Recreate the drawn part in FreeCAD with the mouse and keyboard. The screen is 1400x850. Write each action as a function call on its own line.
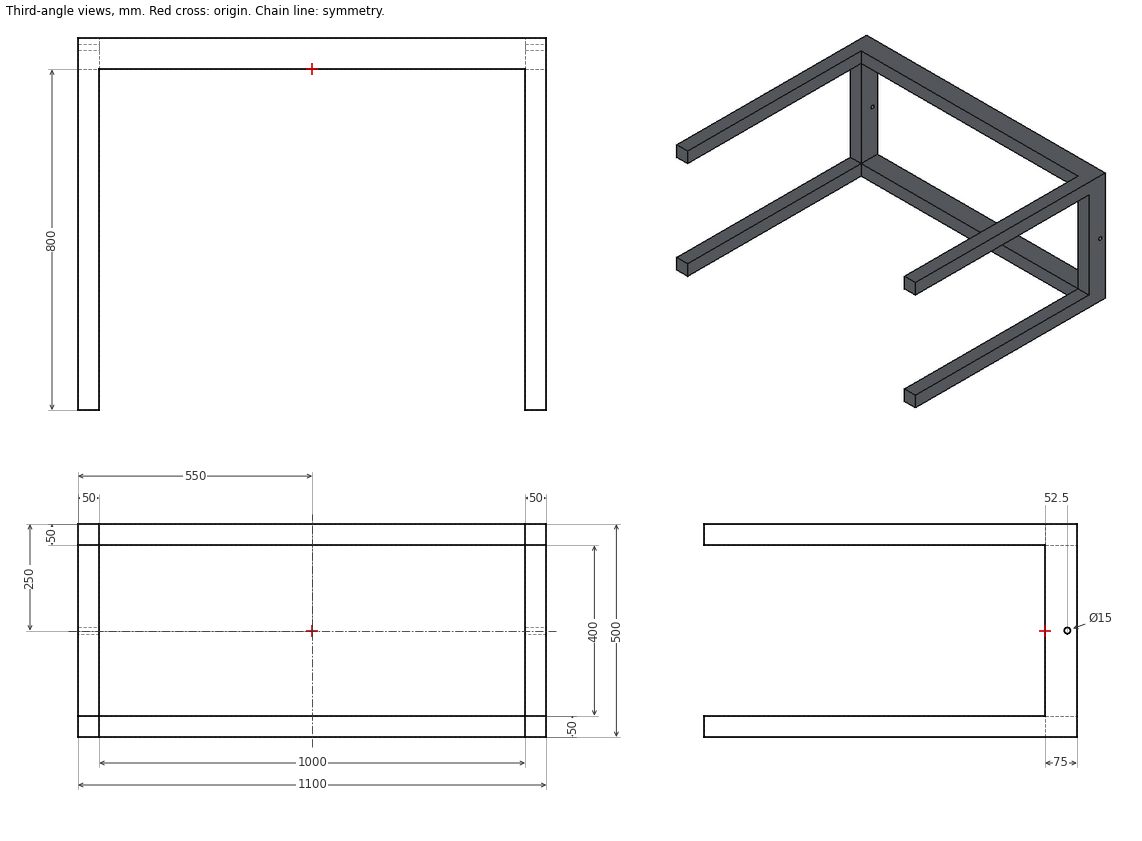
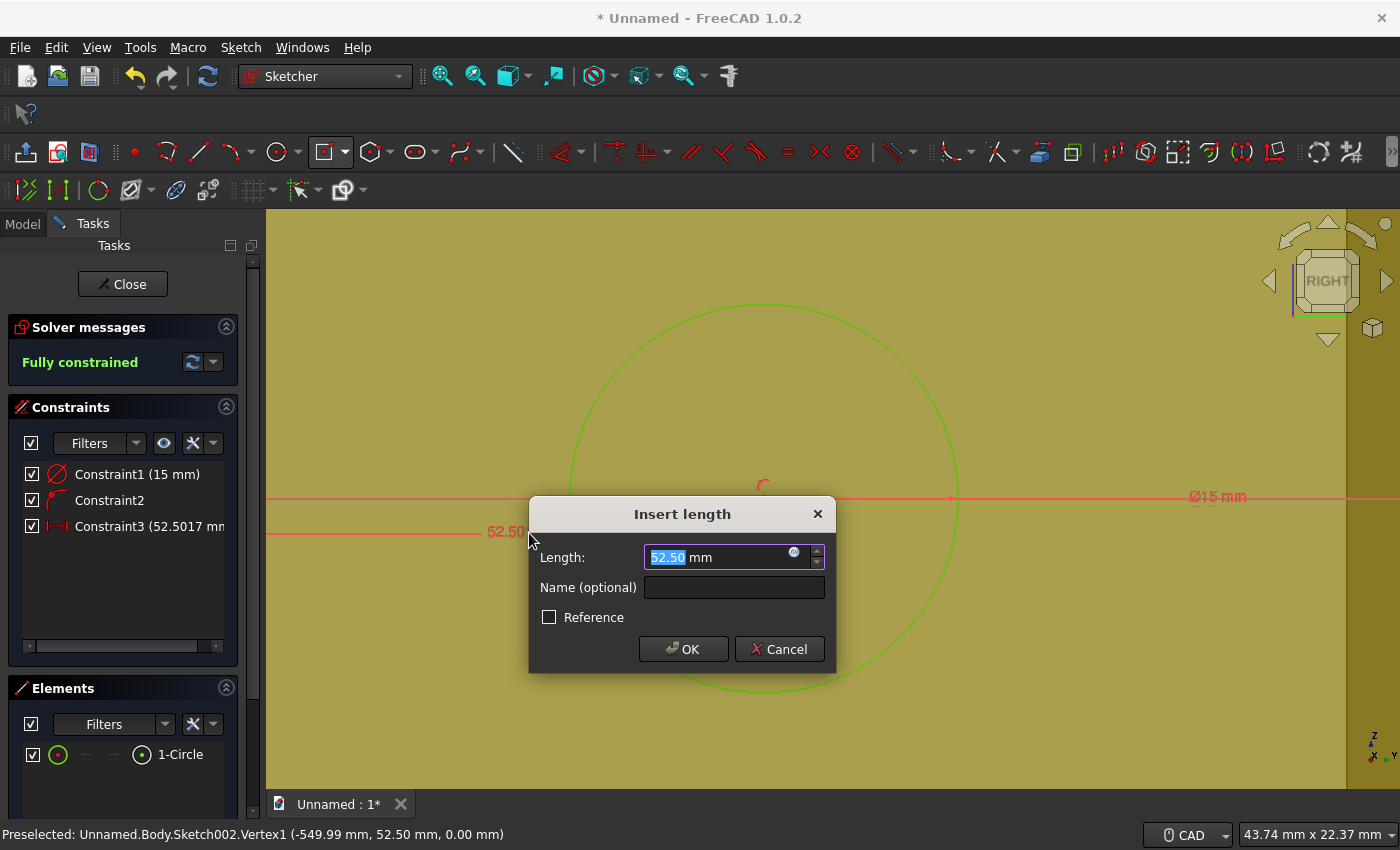
text(52.5)
key(Return)
key(Escape)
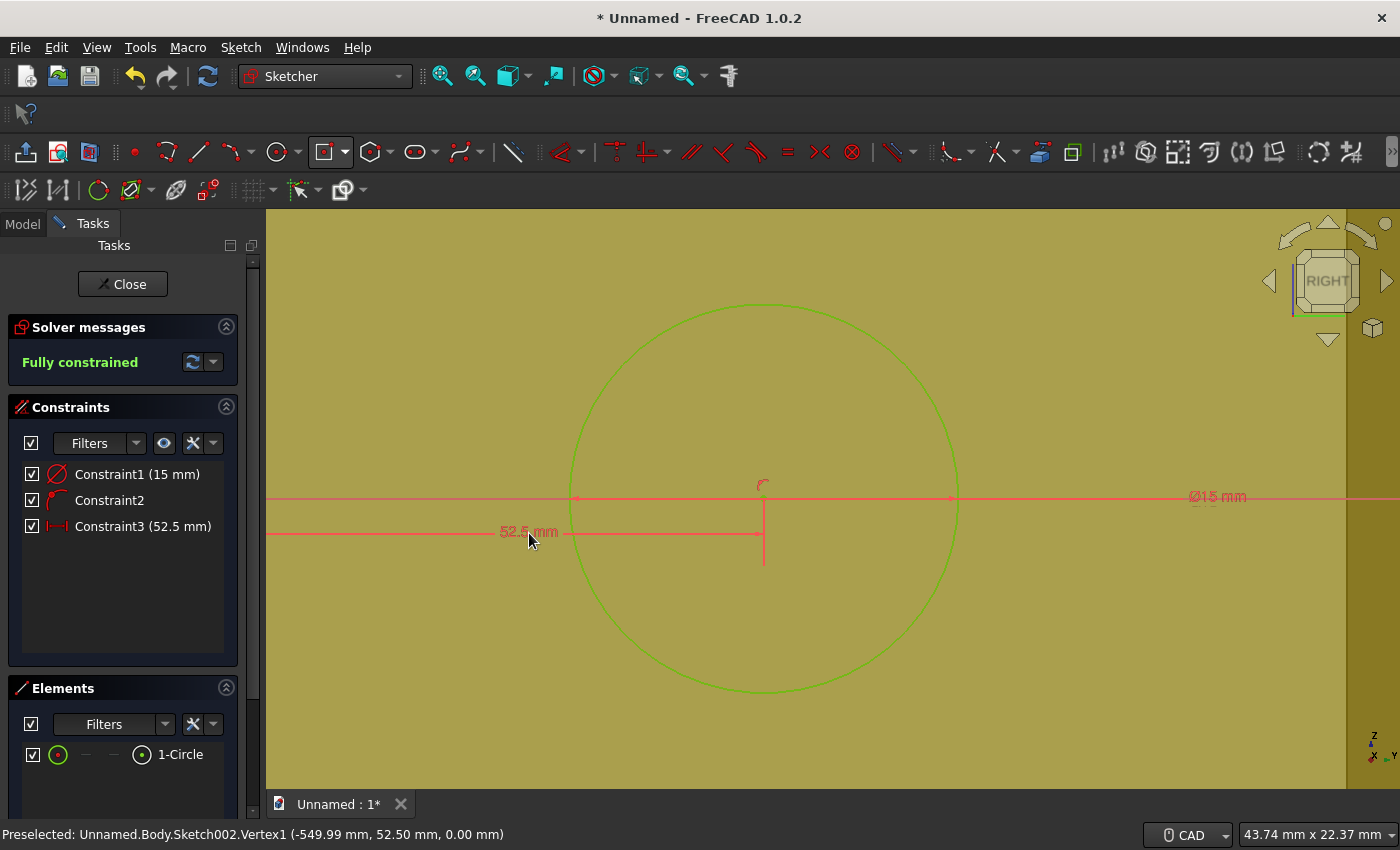
click(123, 284)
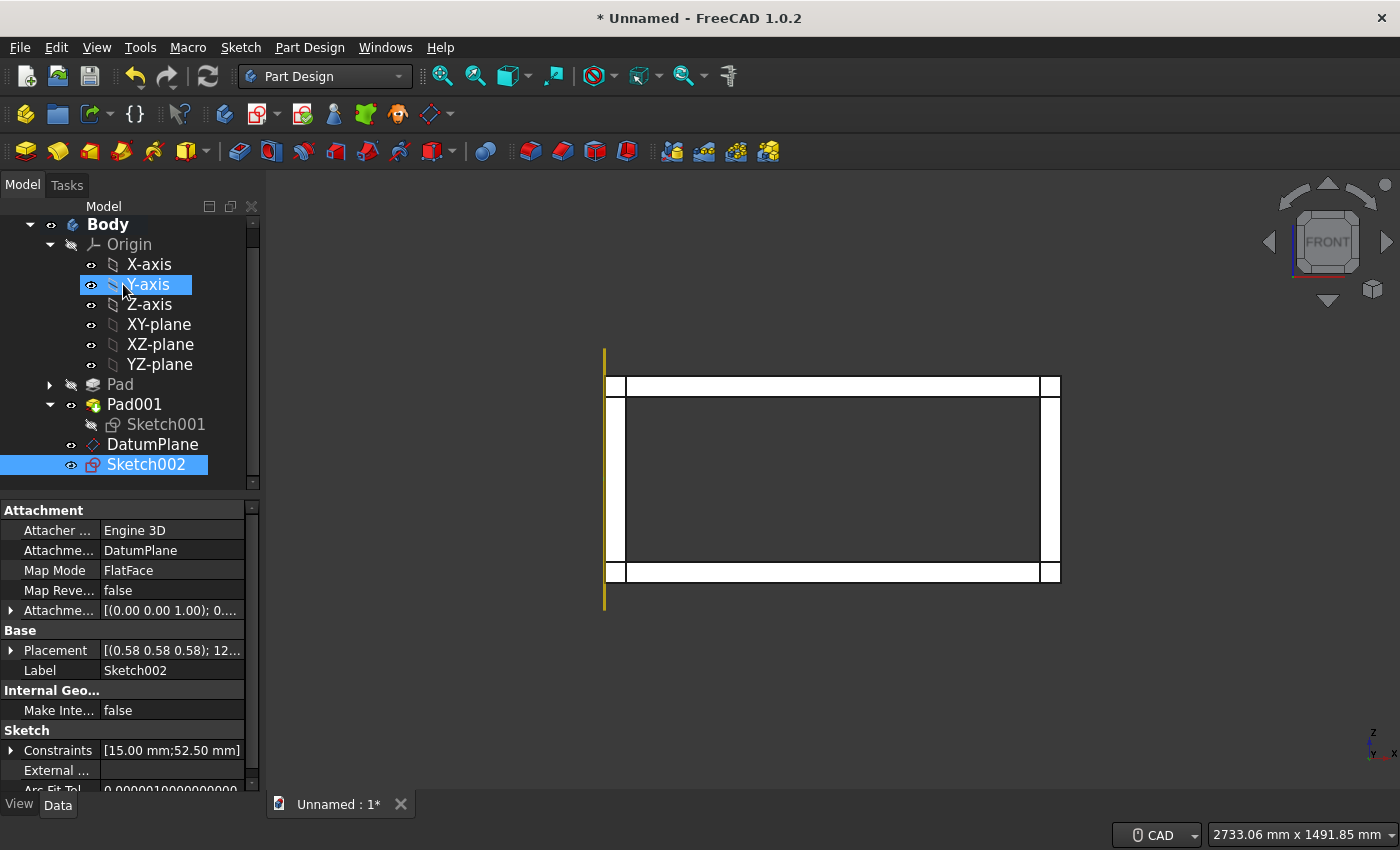
click(240, 152)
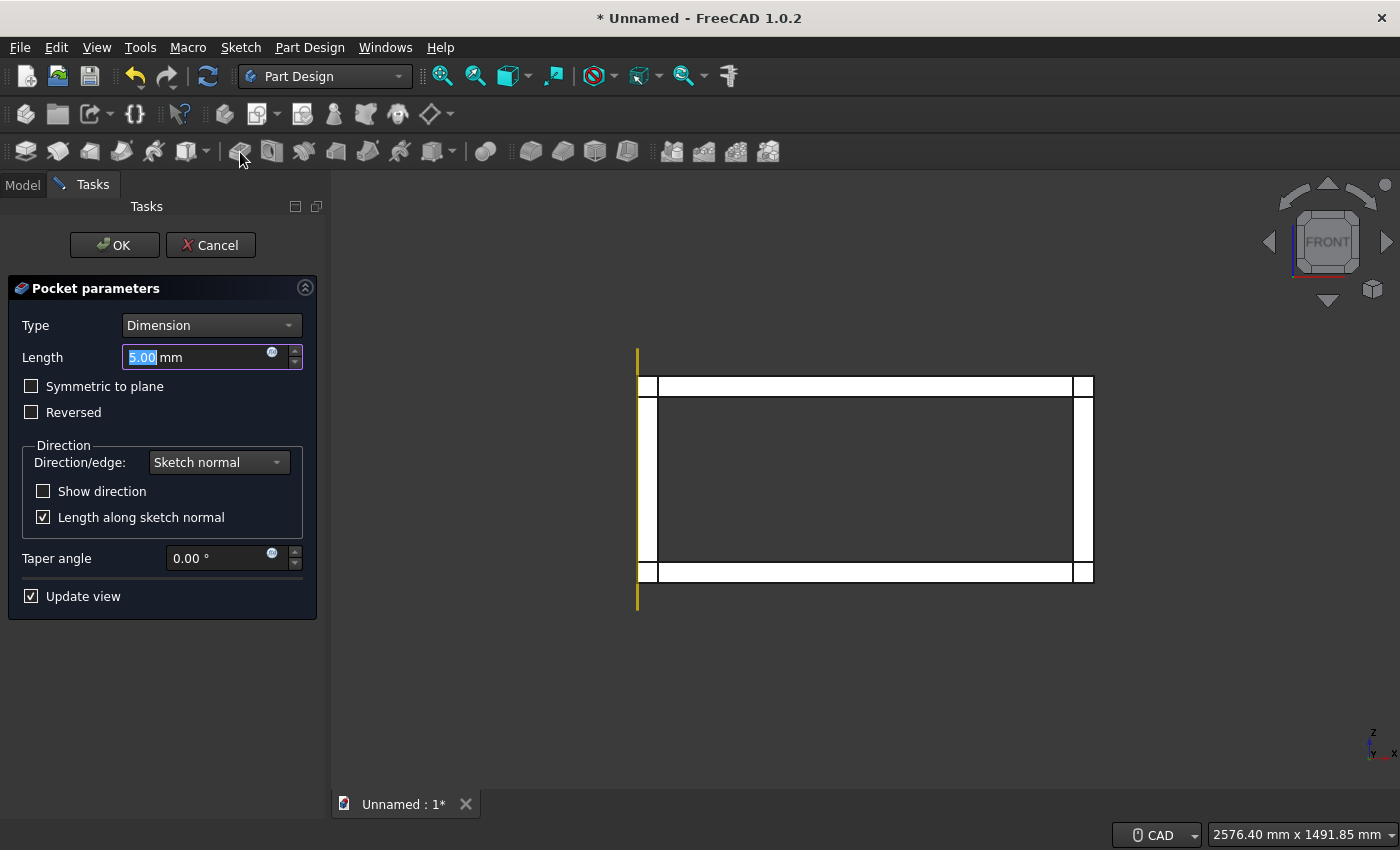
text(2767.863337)
key(Tab)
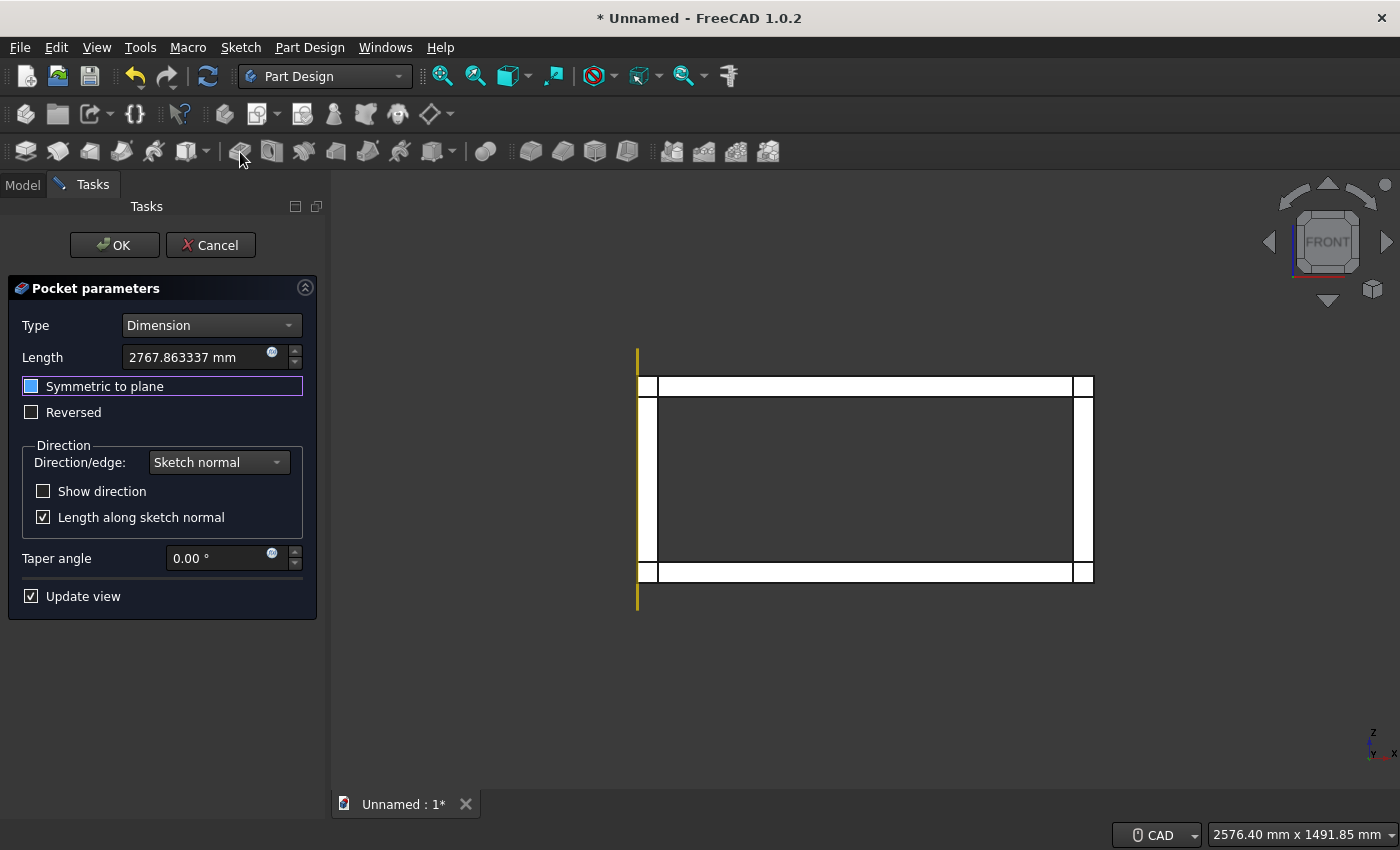
click(30, 386)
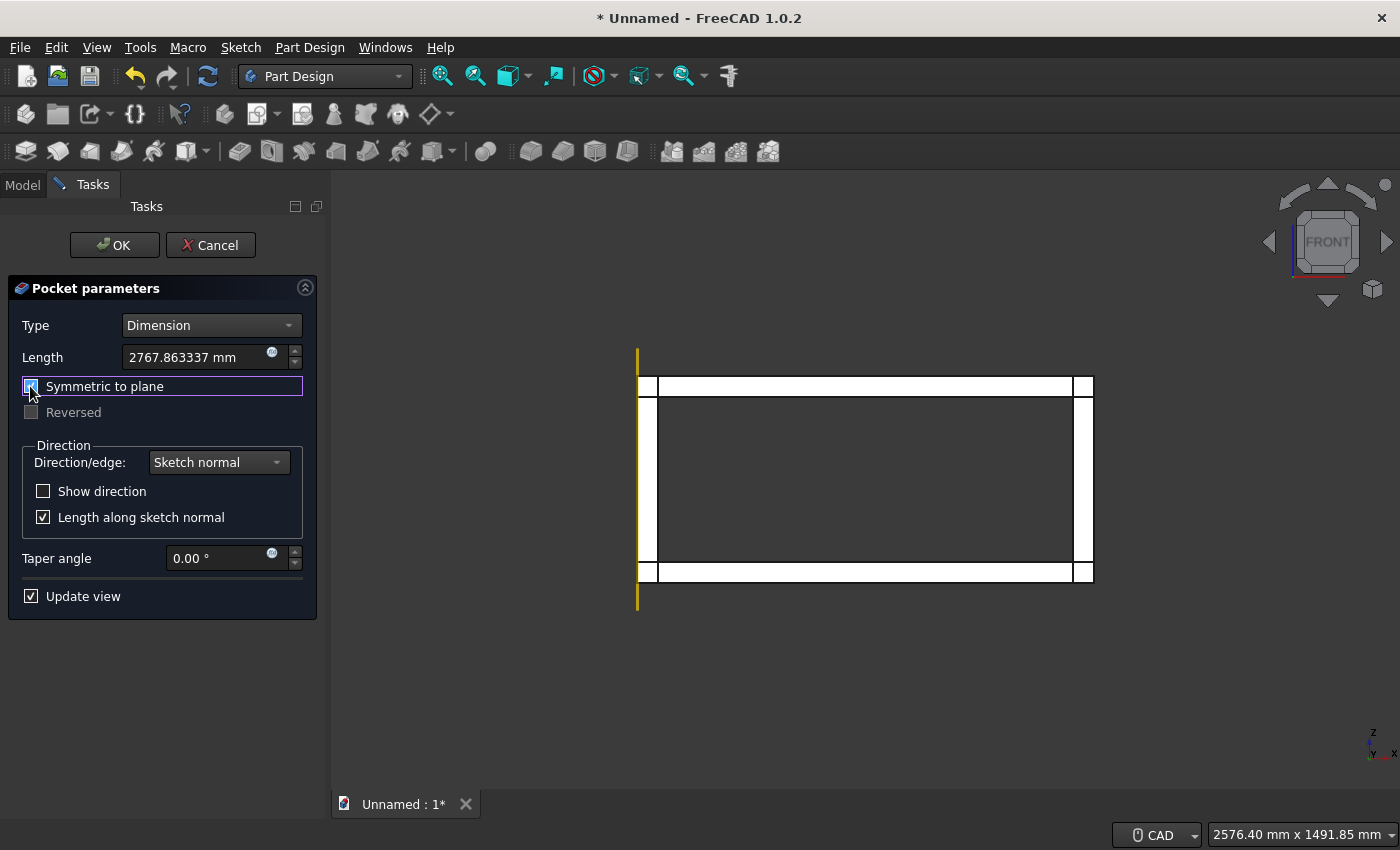
click(115, 245)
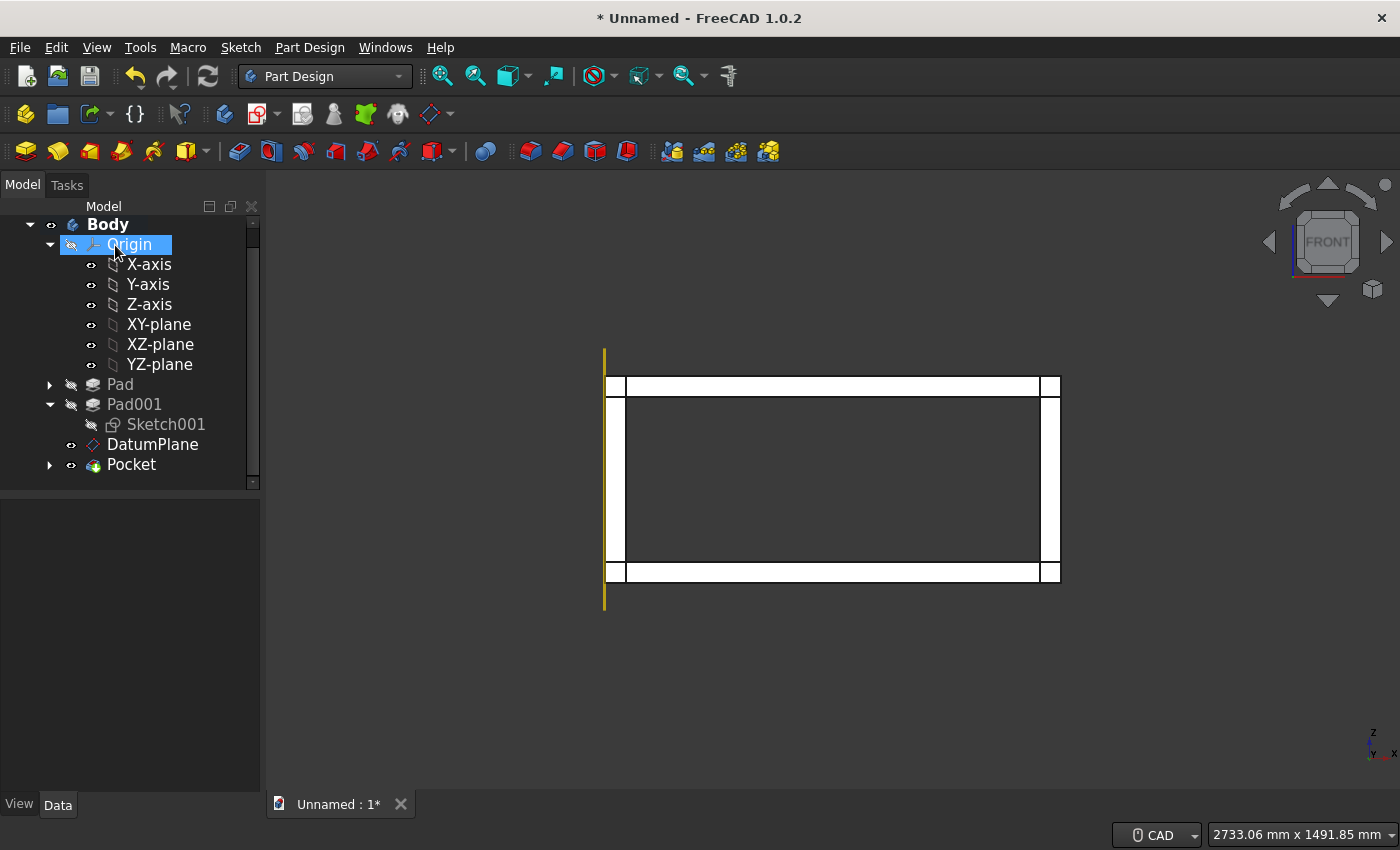
click(116, 445)
key(space)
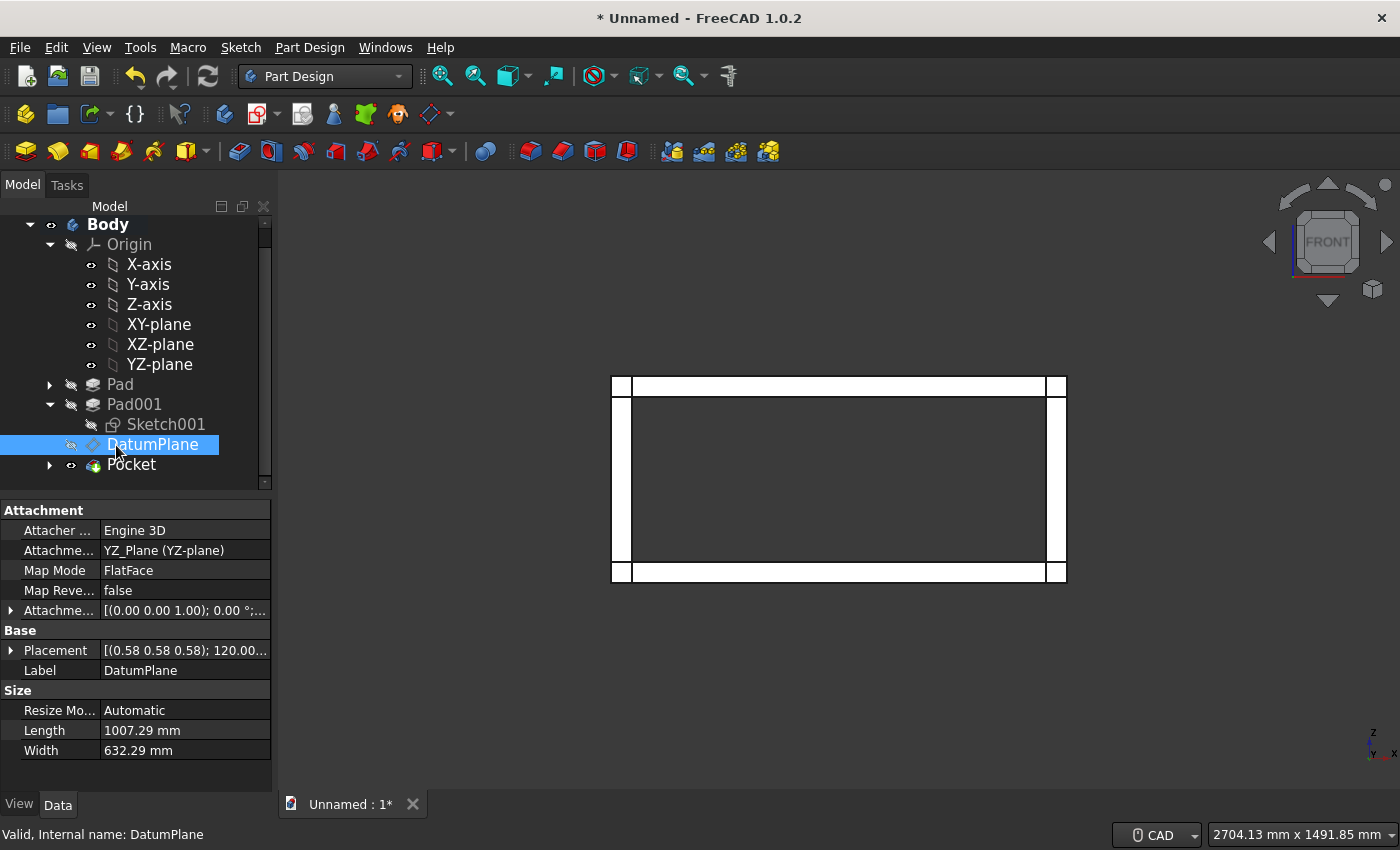
key(0)